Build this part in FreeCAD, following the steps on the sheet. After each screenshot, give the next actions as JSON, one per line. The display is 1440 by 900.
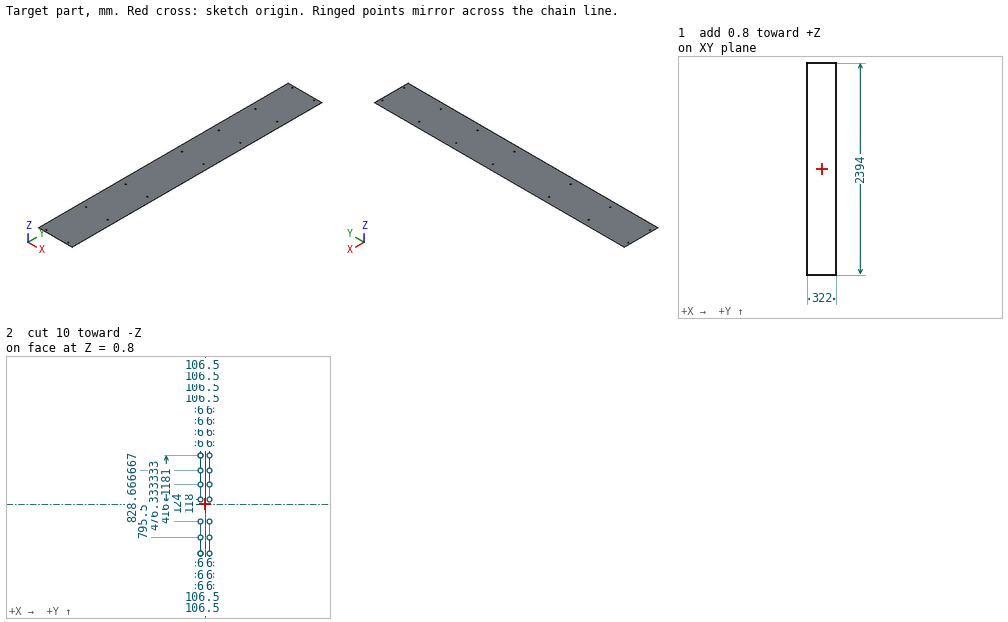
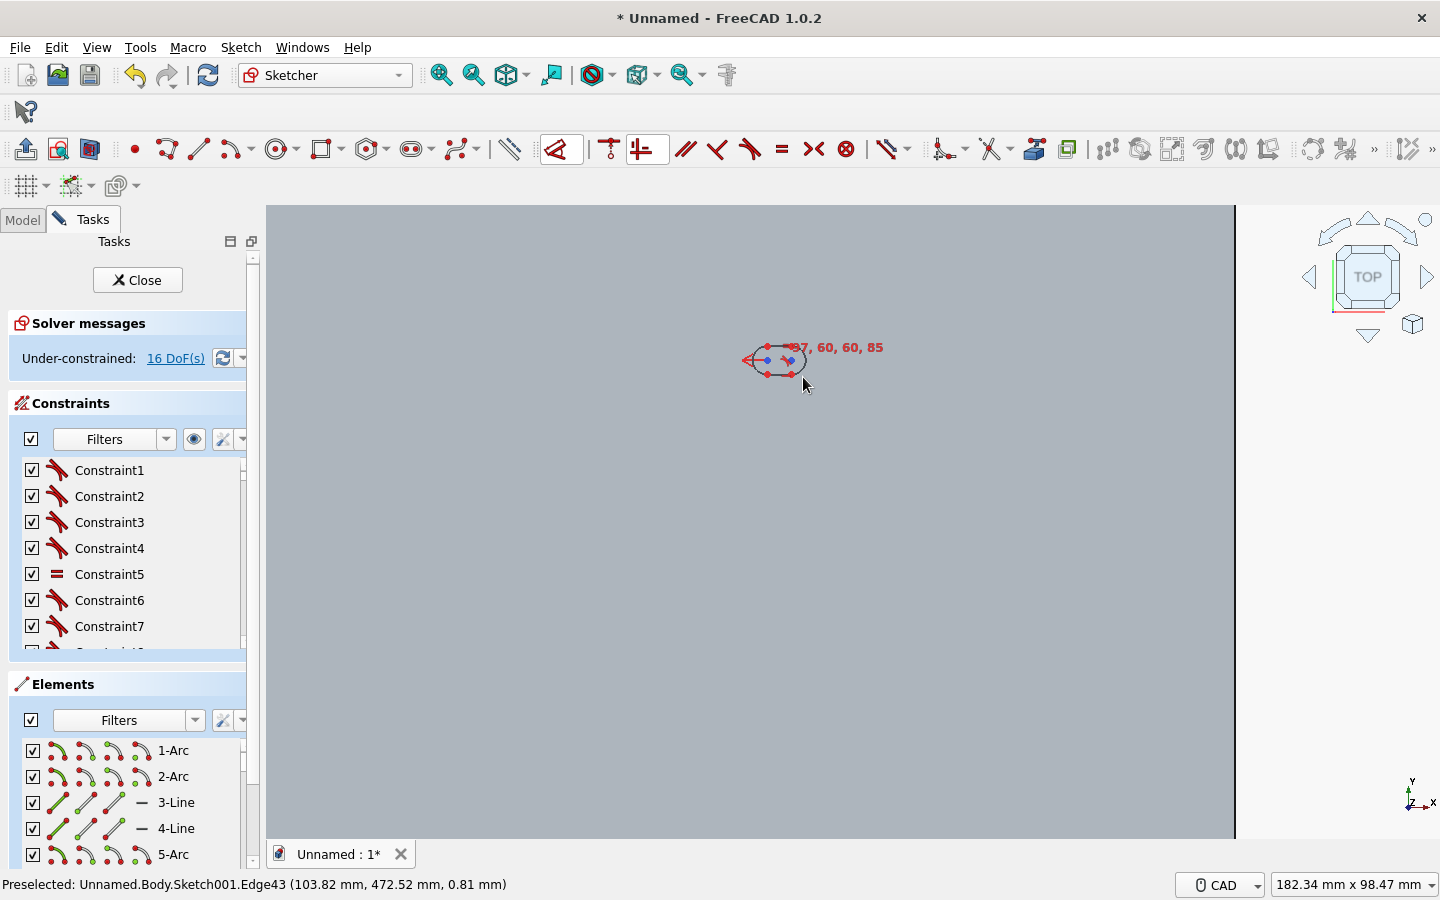
{"action": "left_click", "coordinate": [774, 346]}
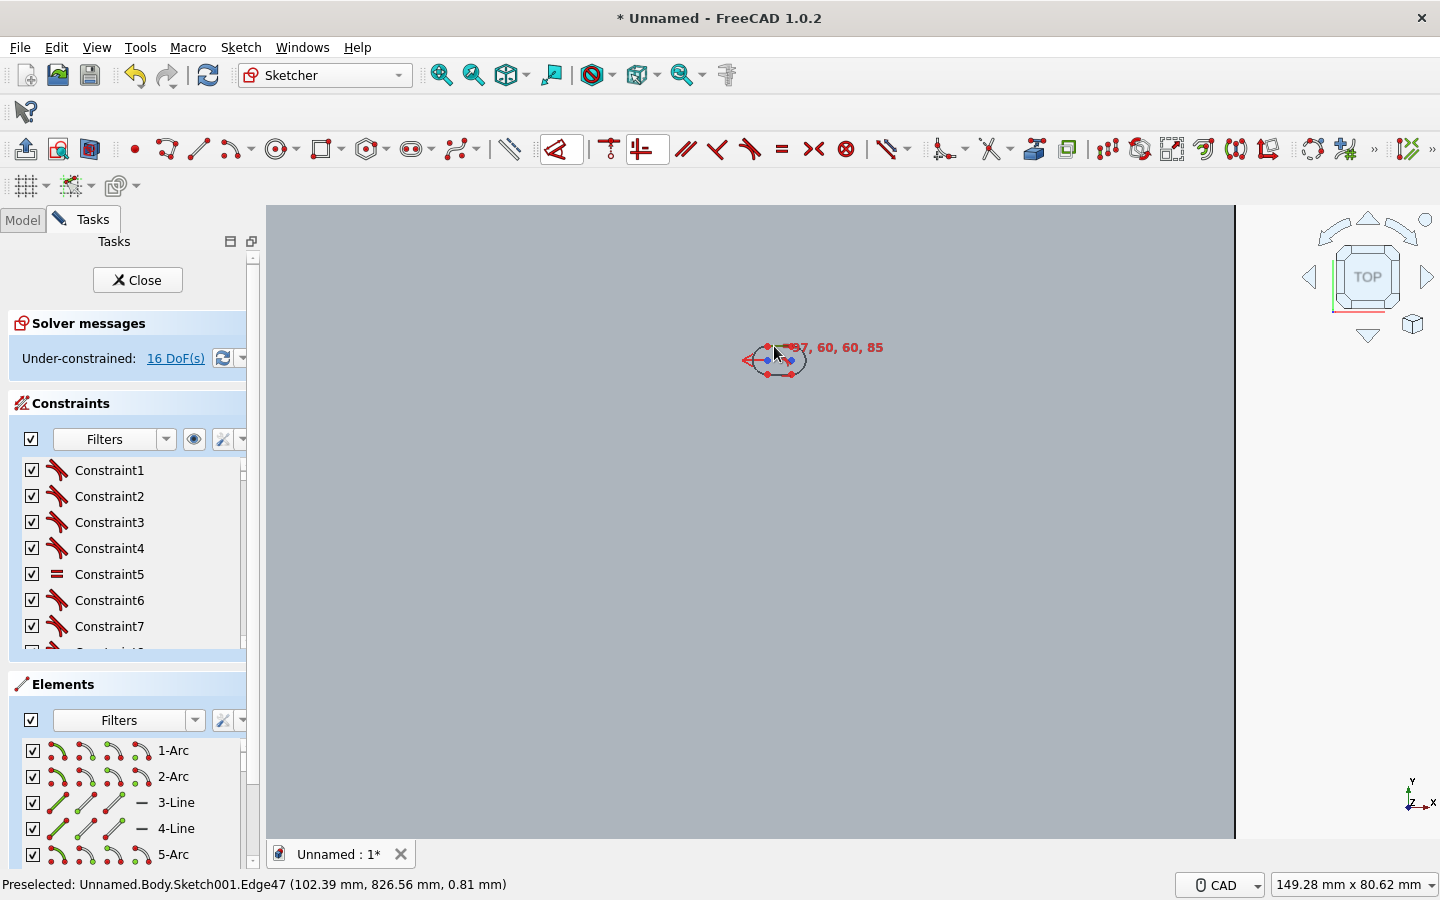
{"action": "key", "text": "l"}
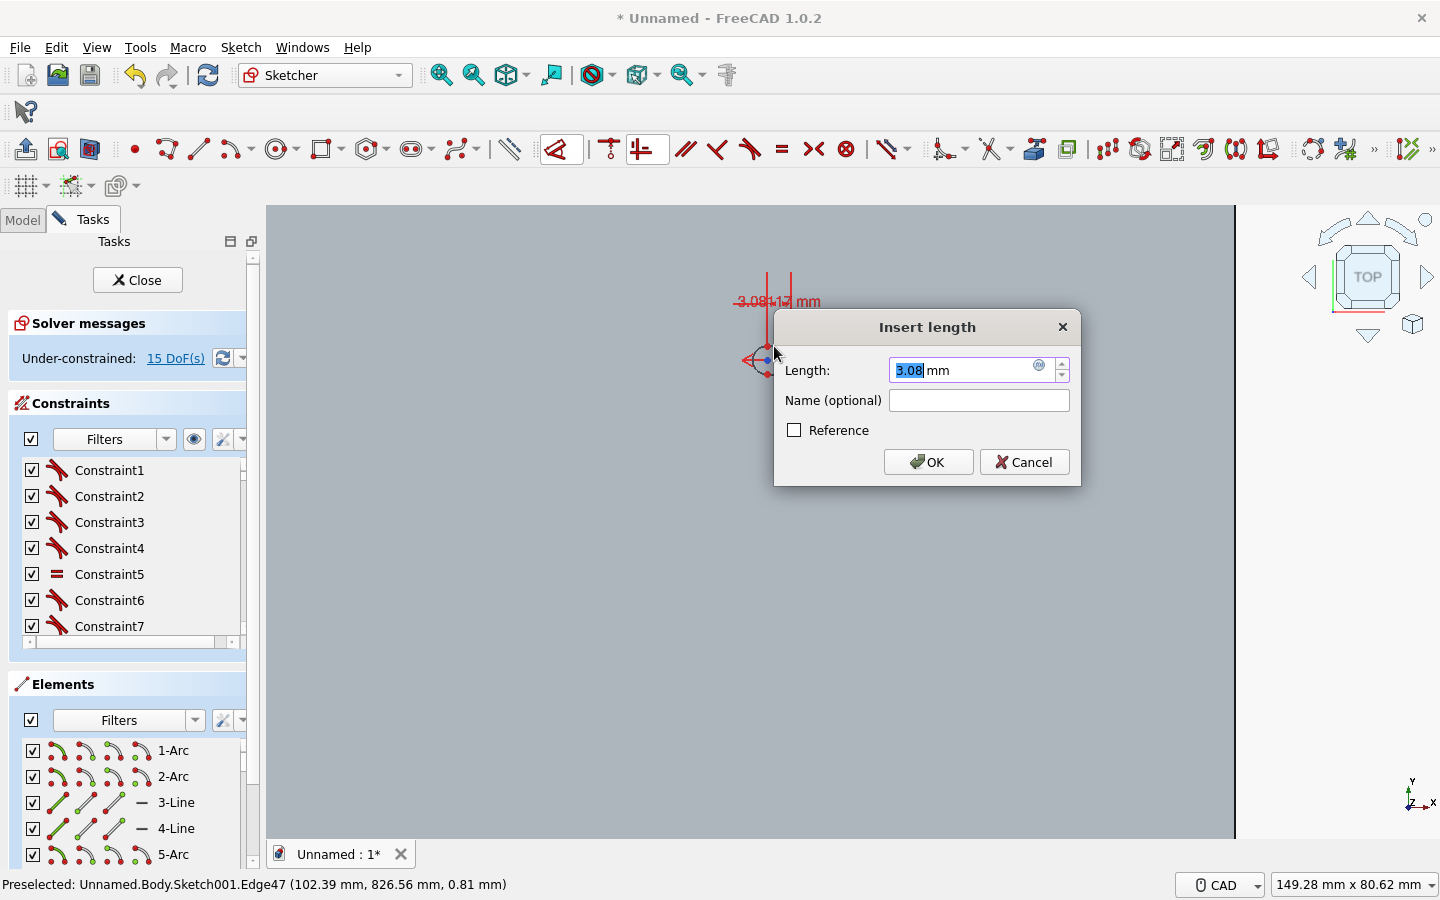
{"action": "type", "text": "6"}
{"action": "key", "text": "Return"}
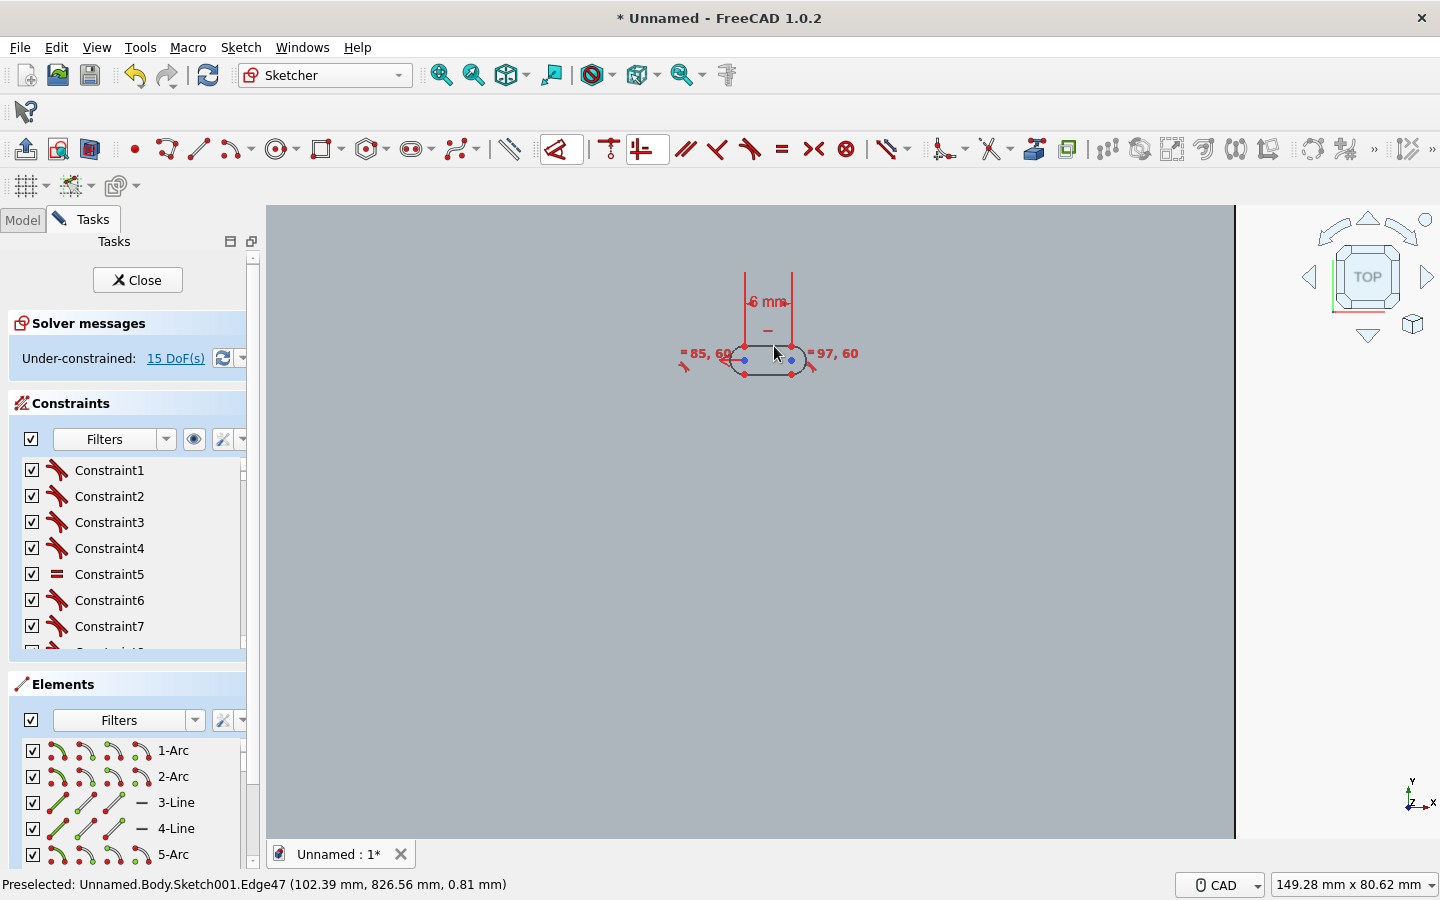
{"action": "scroll", "coordinate": [807, 344], "scroll_direction": "down", "scroll_amount": 18}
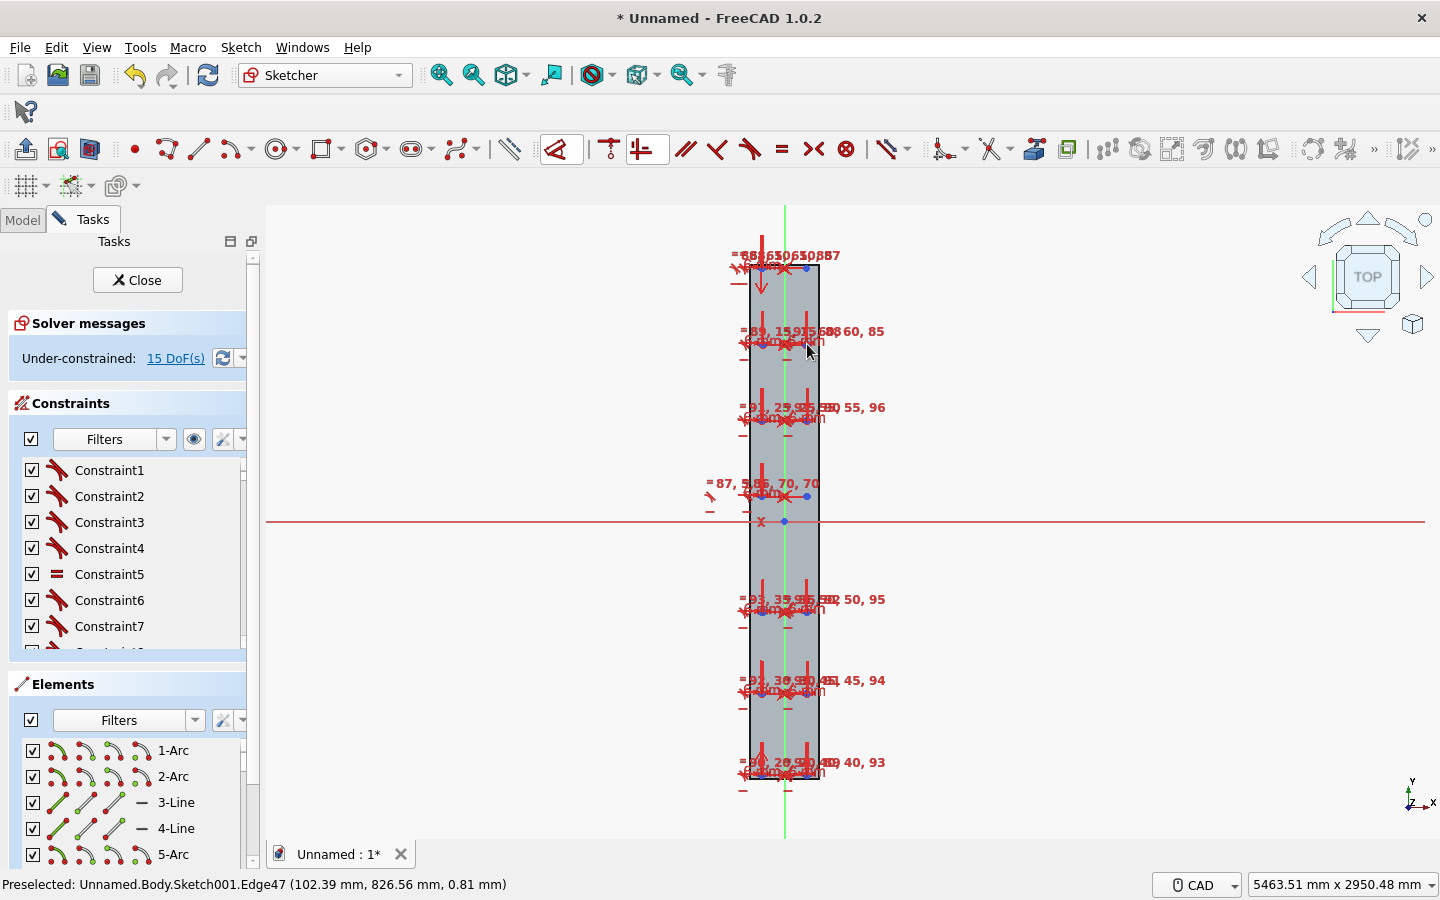
{"action": "scroll", "coordinate": [807, 268], "scroll_direction": "up", "scroll_amount": 18}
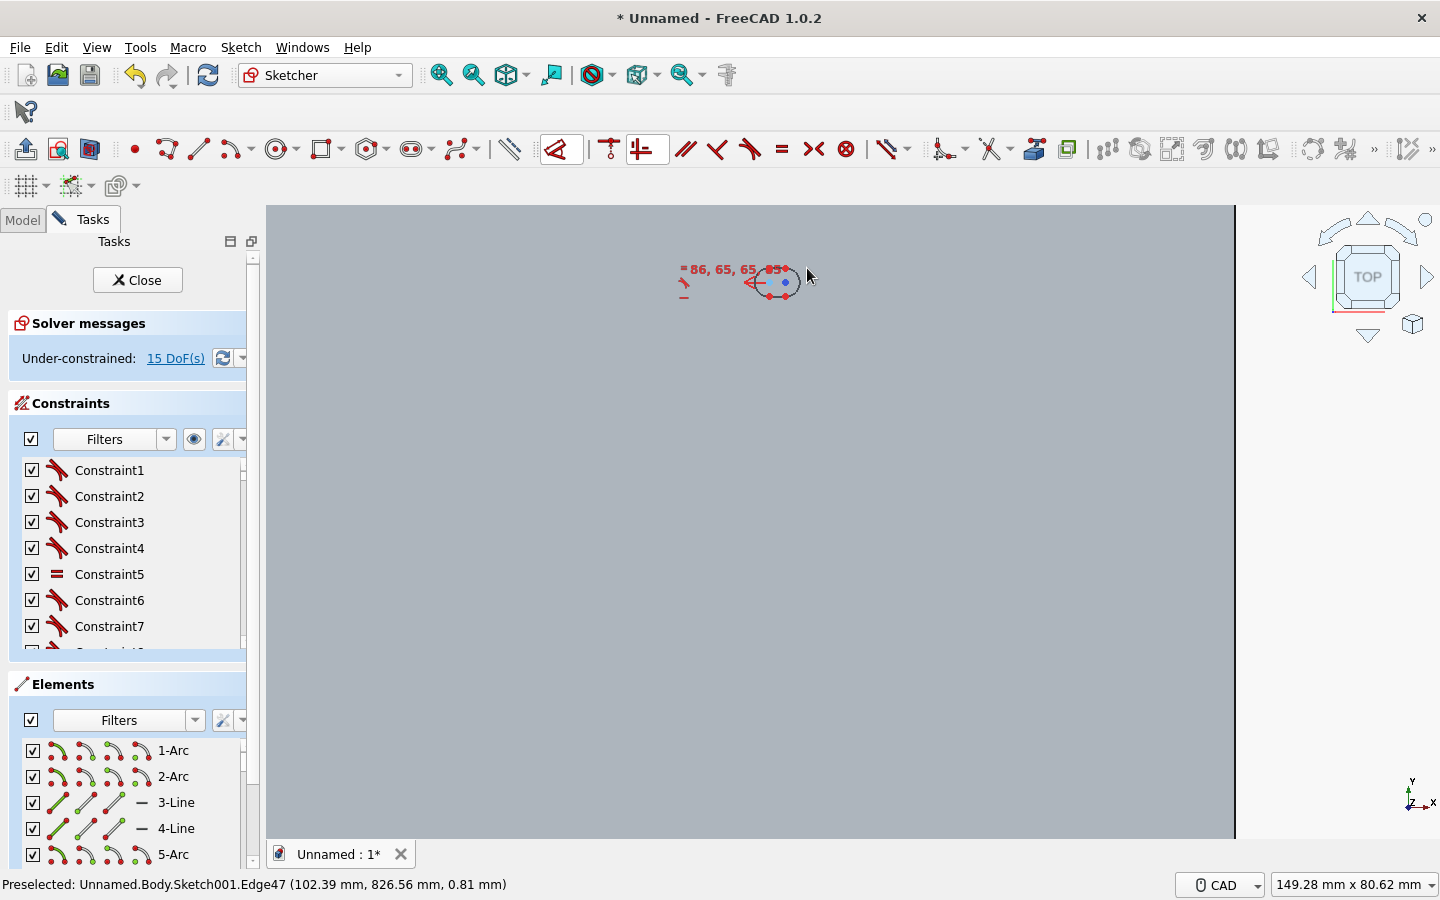
{"action": "scroll", "coordinate": [777, 268], "scroll_direction": "up", "scroll_amount": 4}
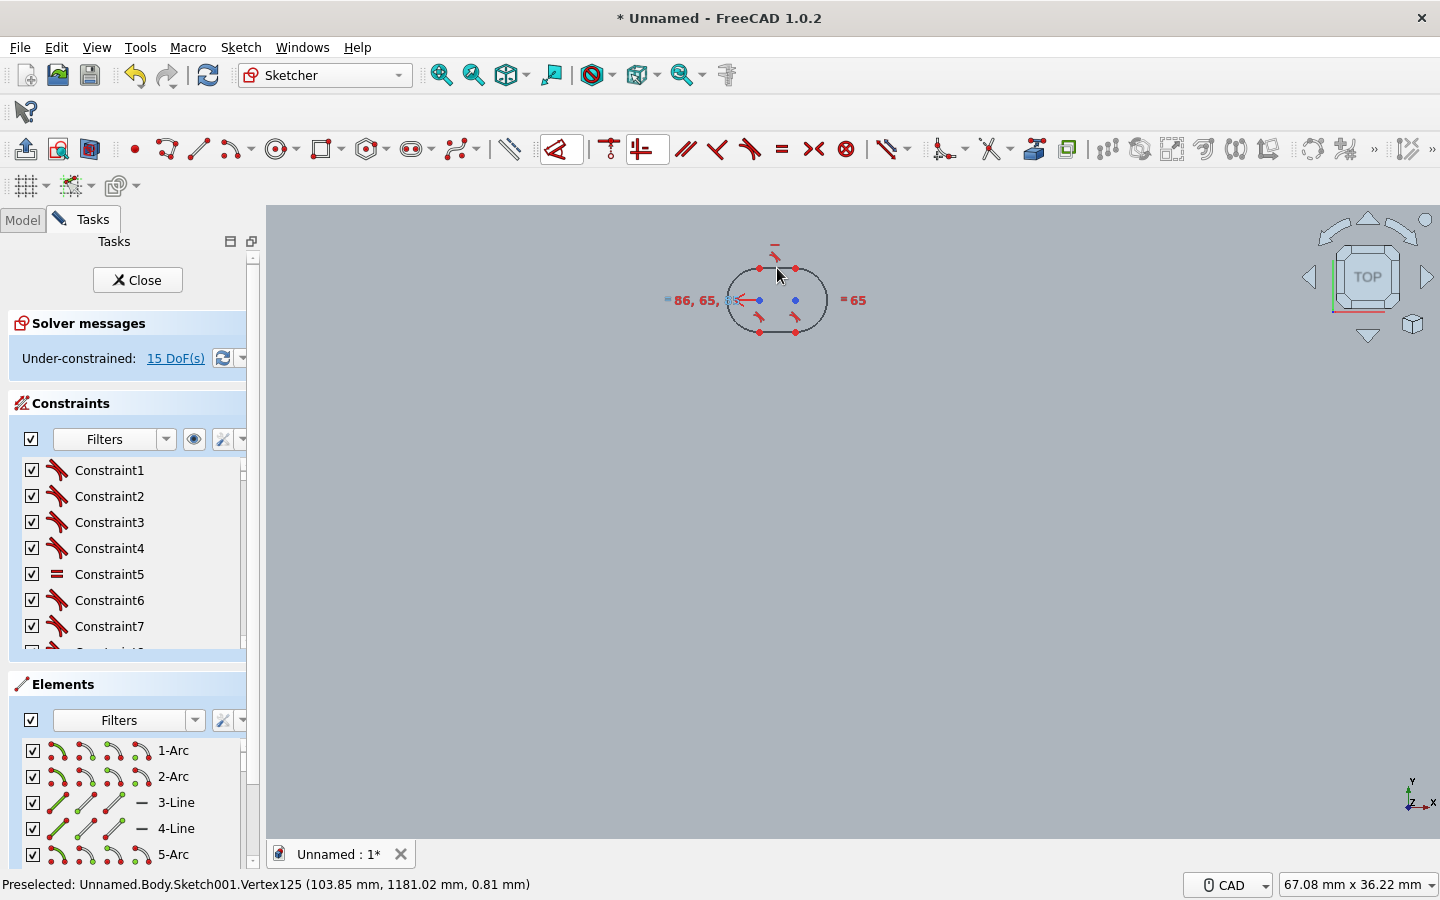
{"action": "left_click", "coordinate": [777, 268]}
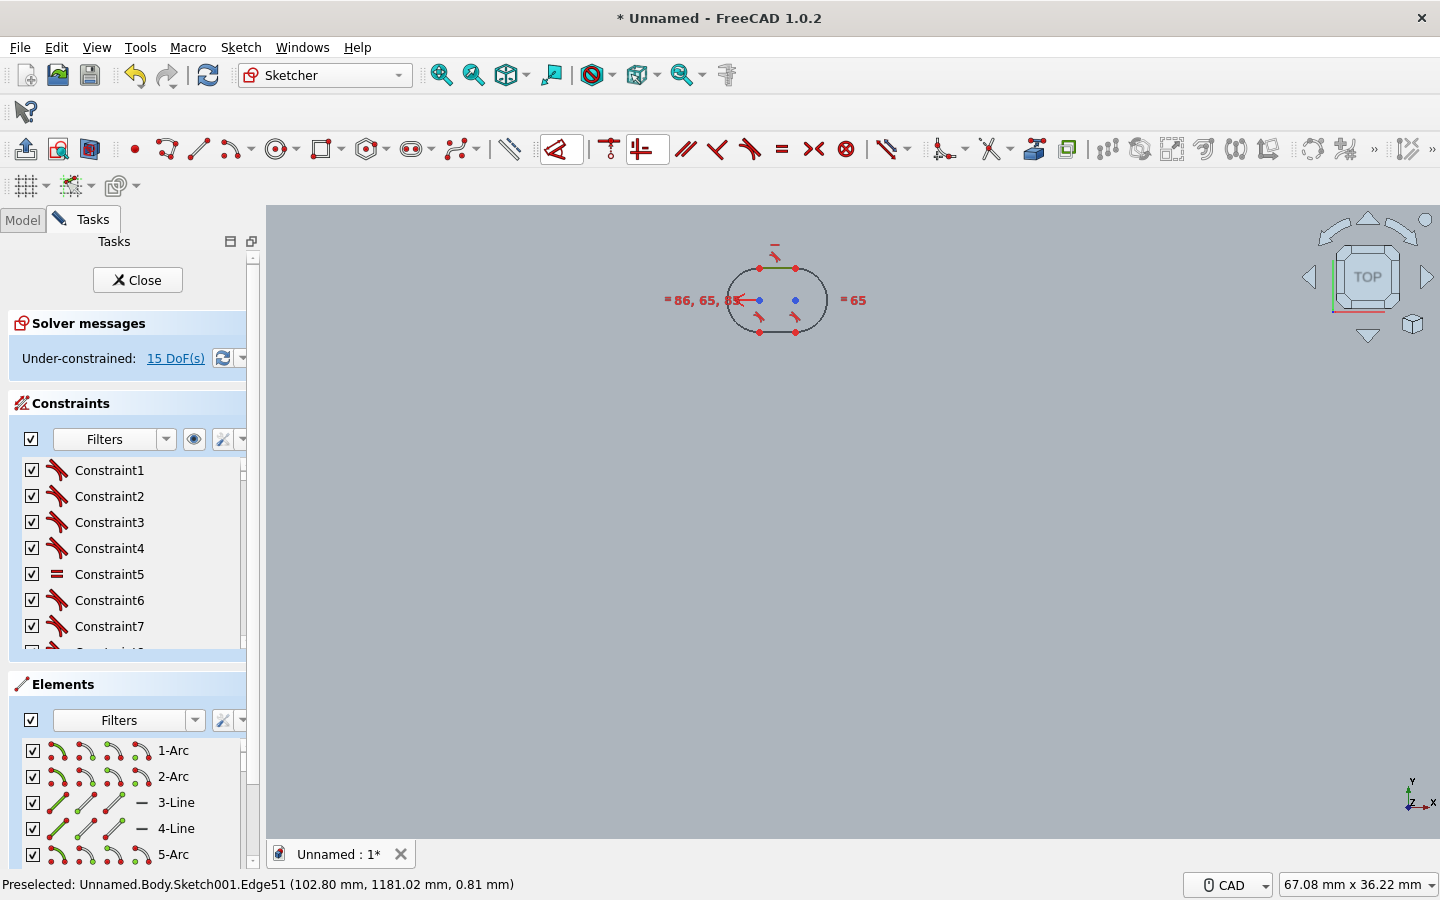
{"action": "key", "text": "l"}